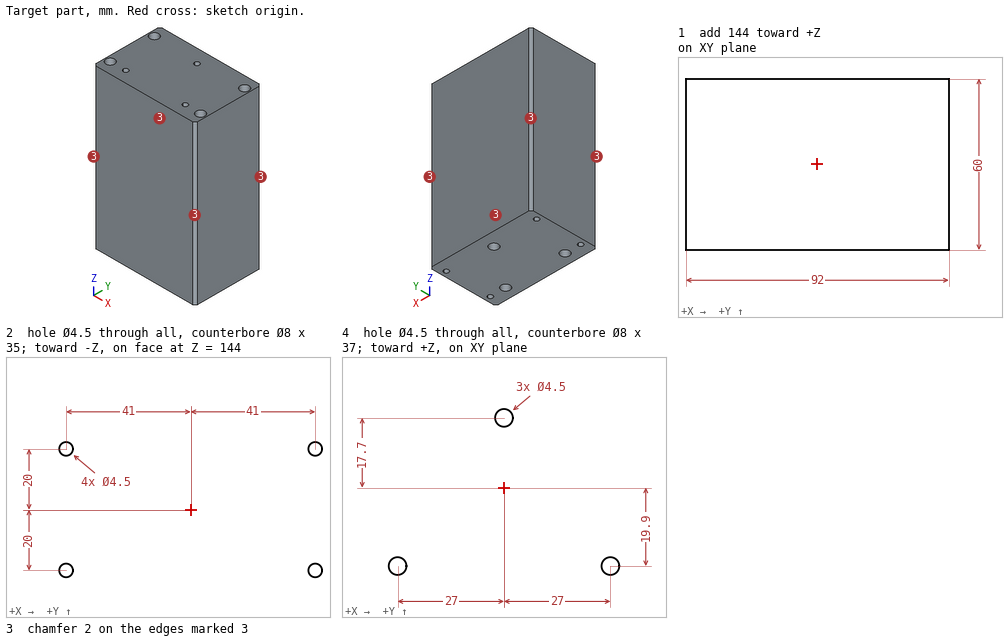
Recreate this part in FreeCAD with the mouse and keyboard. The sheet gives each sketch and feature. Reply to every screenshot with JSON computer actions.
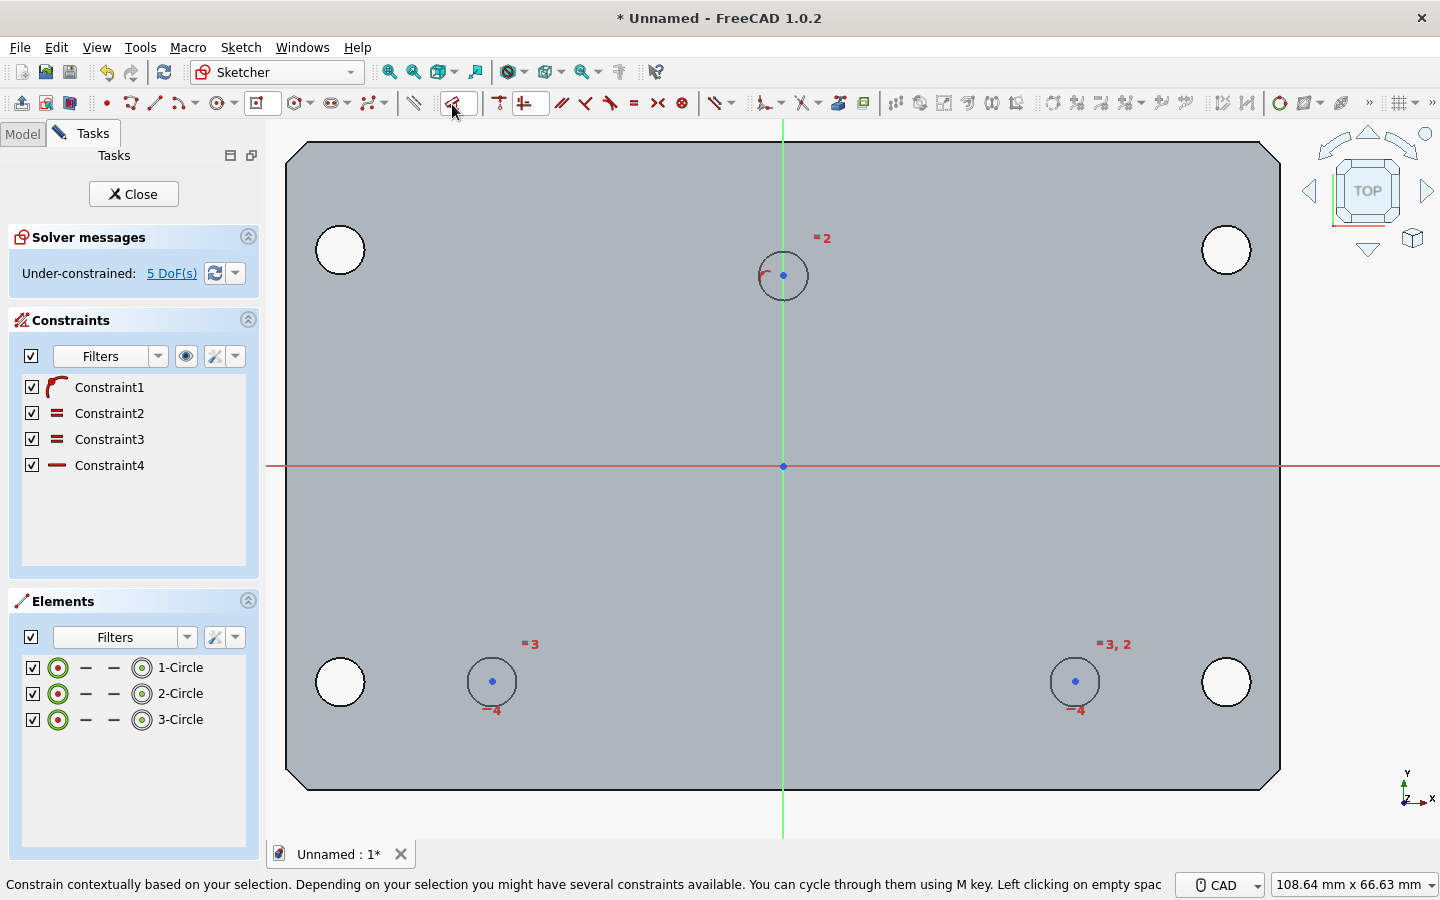
{"action": "left_click", "coordinate": [801, 259]}
{"action": "left_click", "coordinate": [824, 237]}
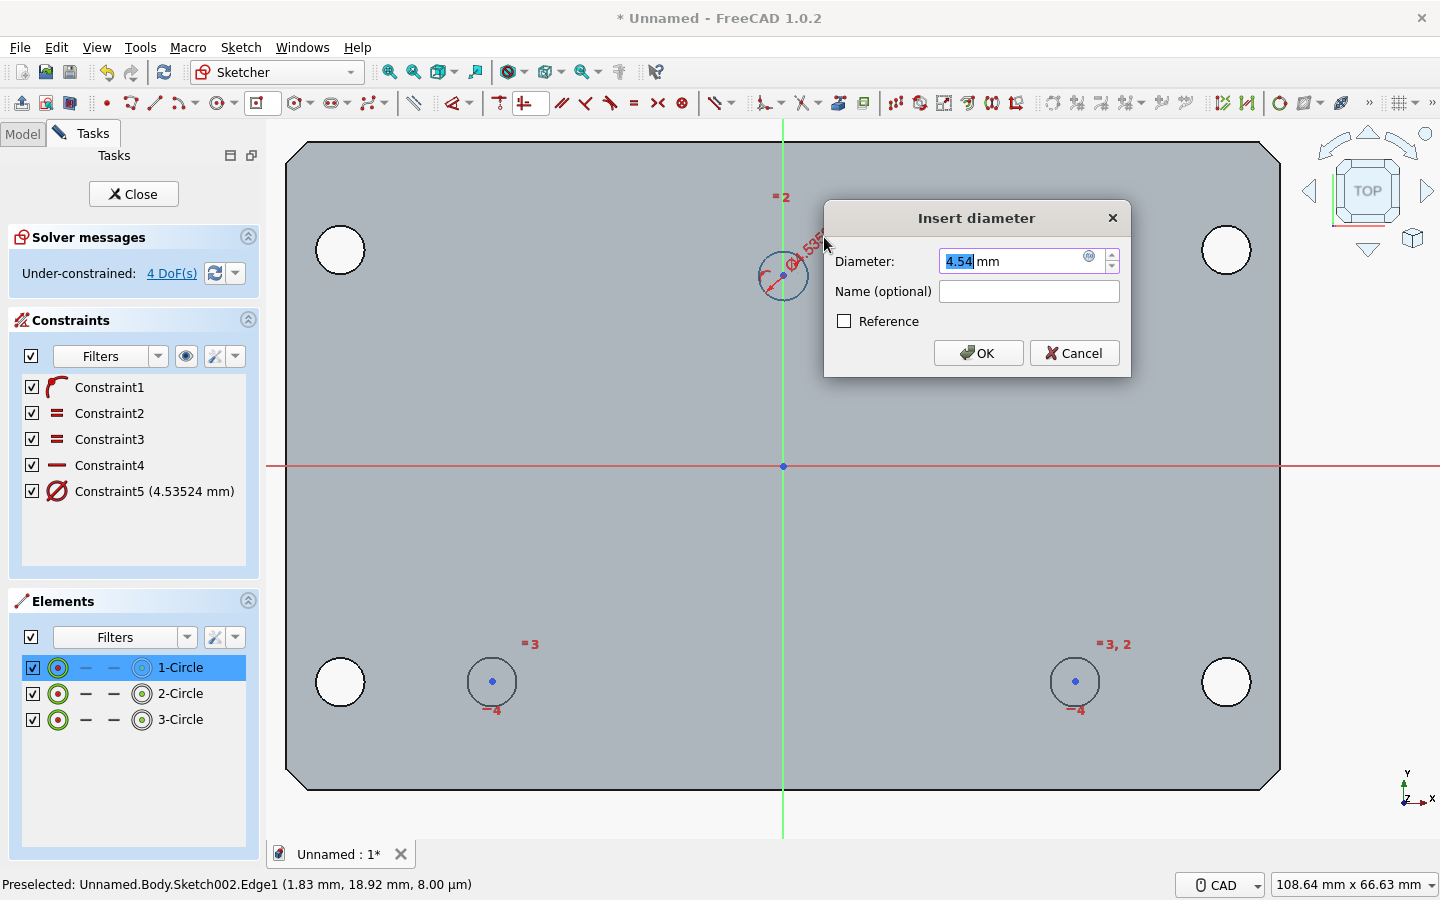
{"action": "type", "text": "4.5"}
{"action": "key", "text": "Return"}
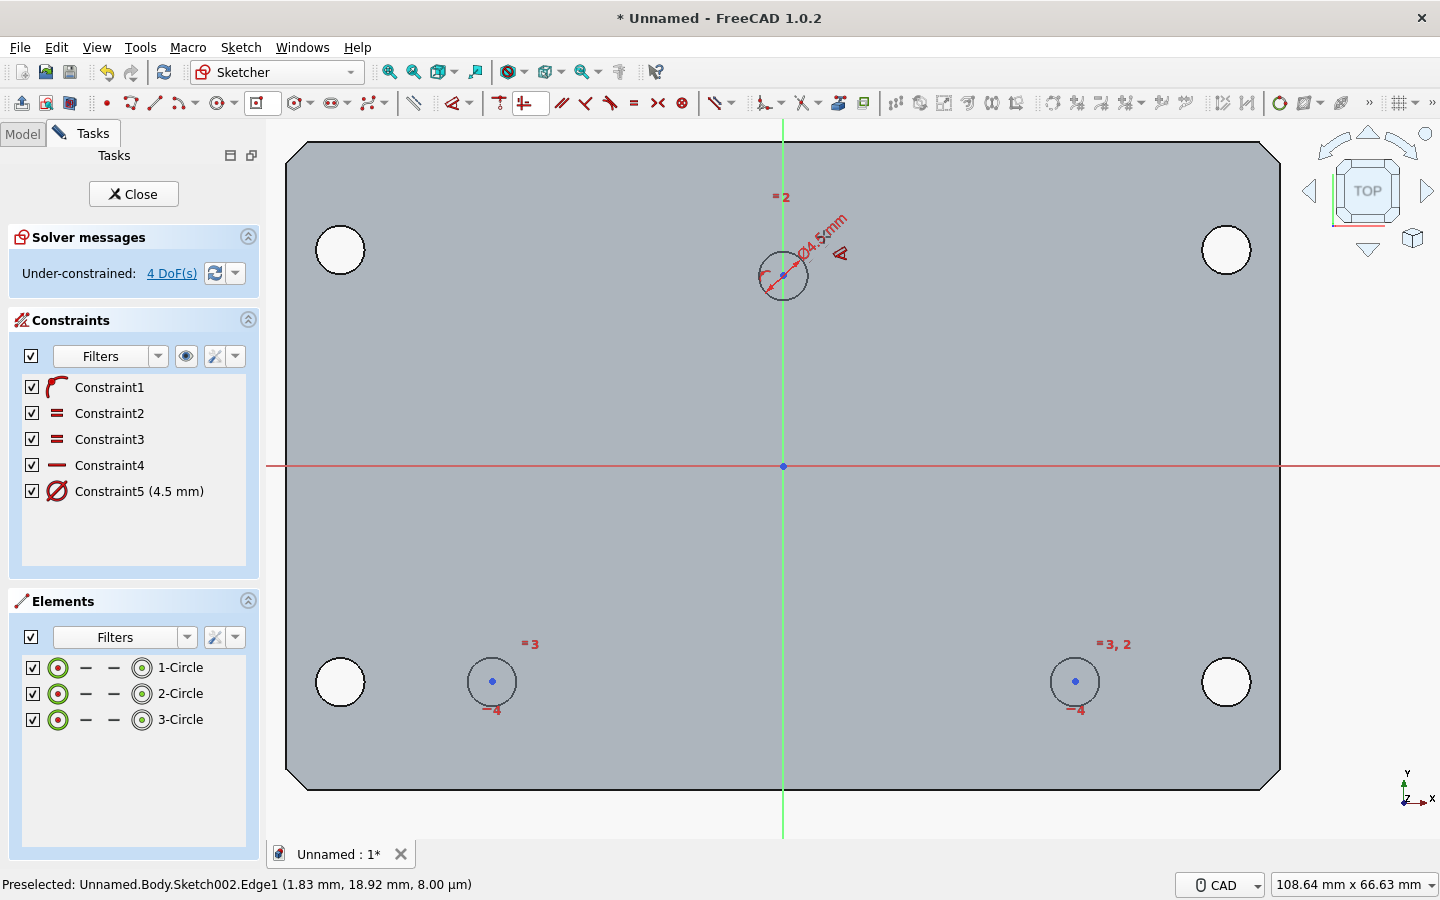
{"action": "left_click", "coordinate": [1075, 682]}
{"action": "left_click", "coordinate": [929, 716]}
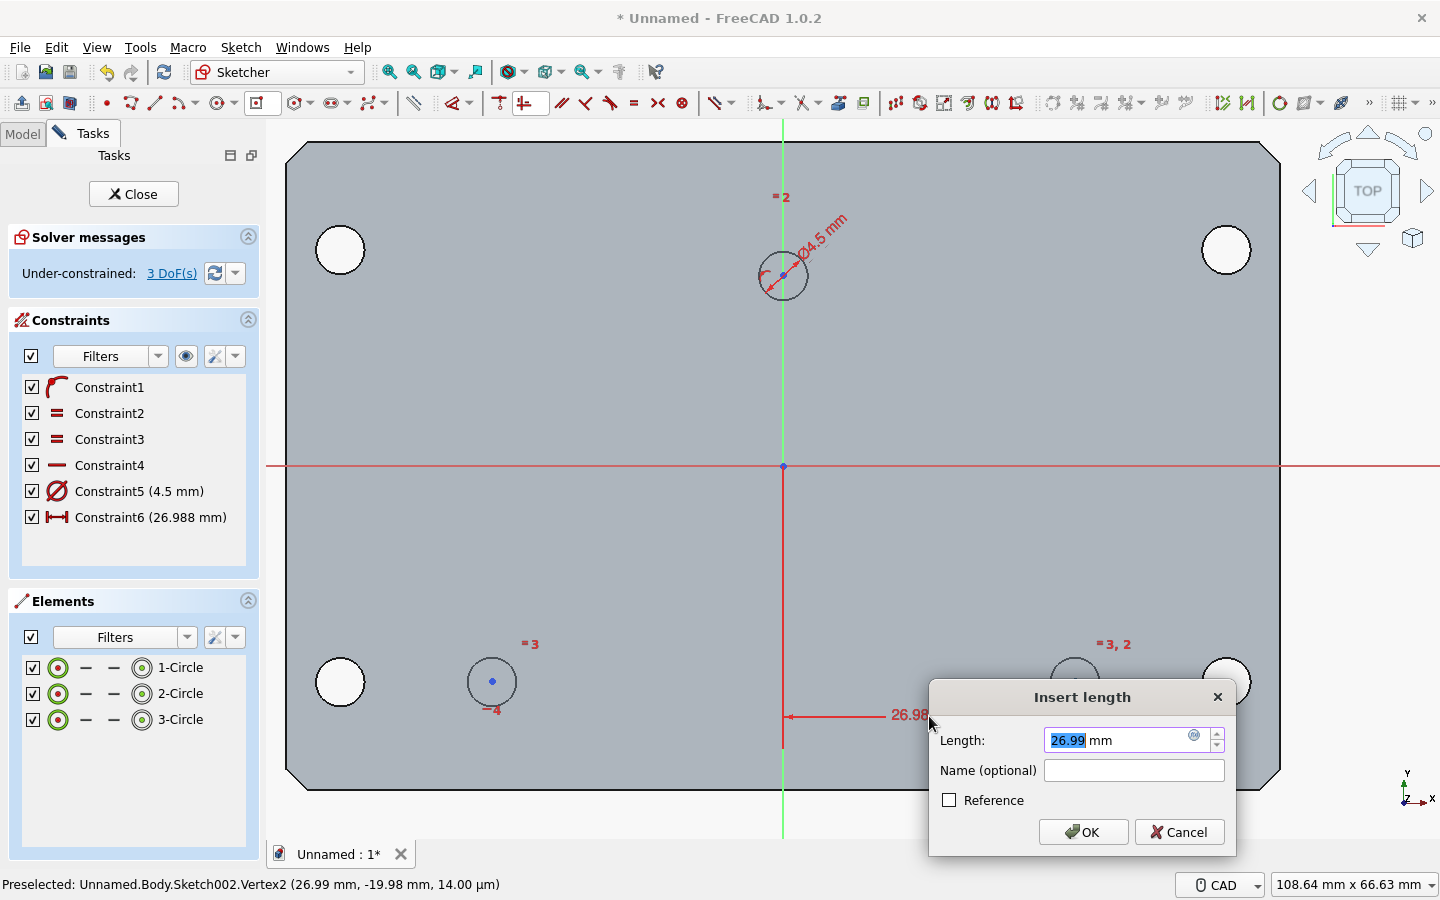
{"action": "type", "text": "27"}
{"action": "key", "text": "Return"}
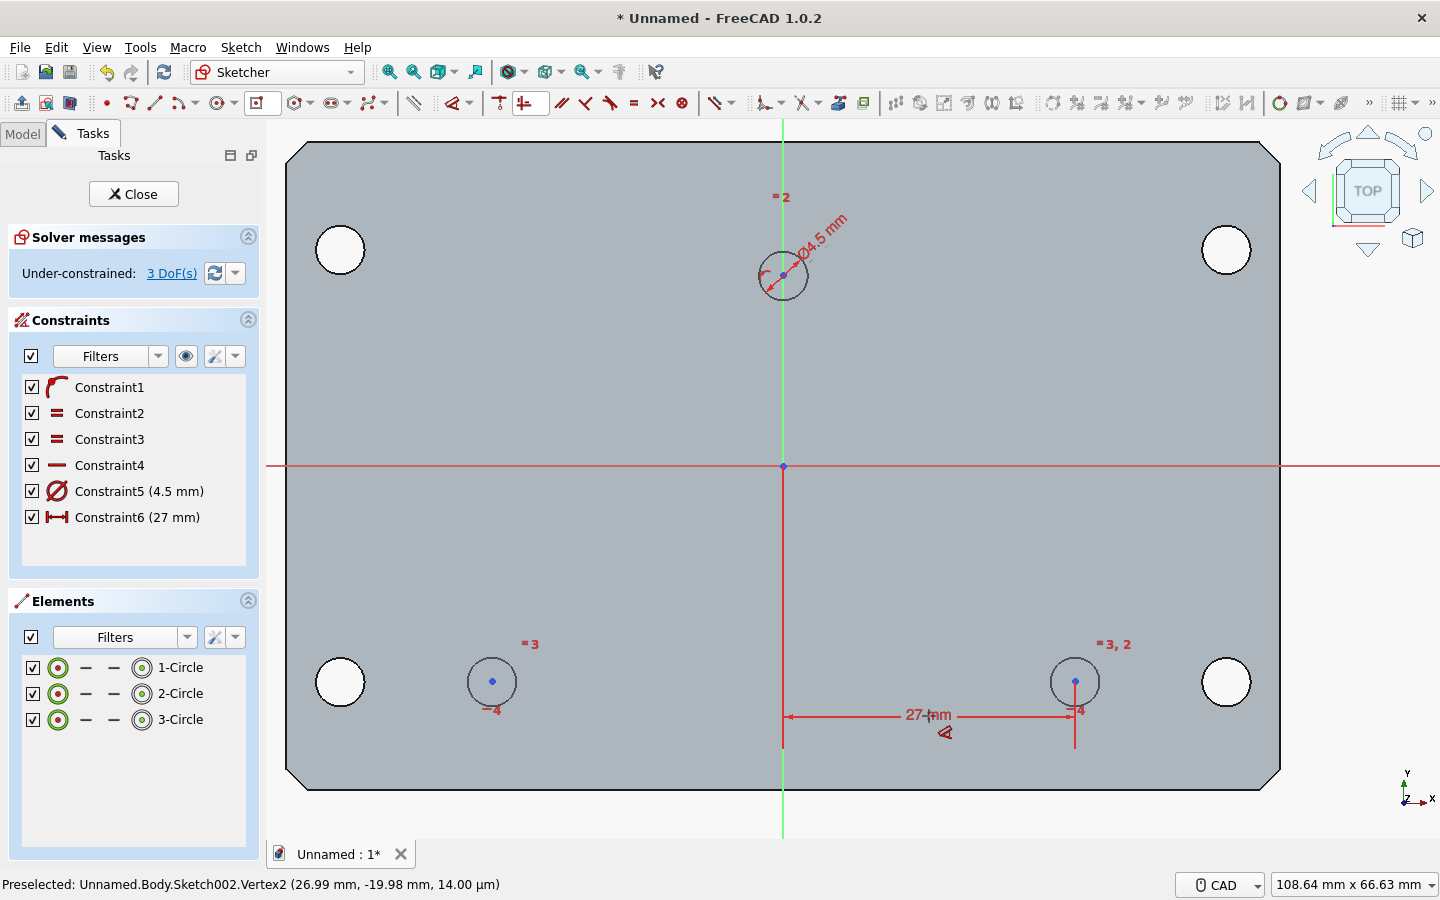
{"action": "left_click", "coordinate": [492, 682]}
{"action": "left_click", "coordinate": [638, 716]}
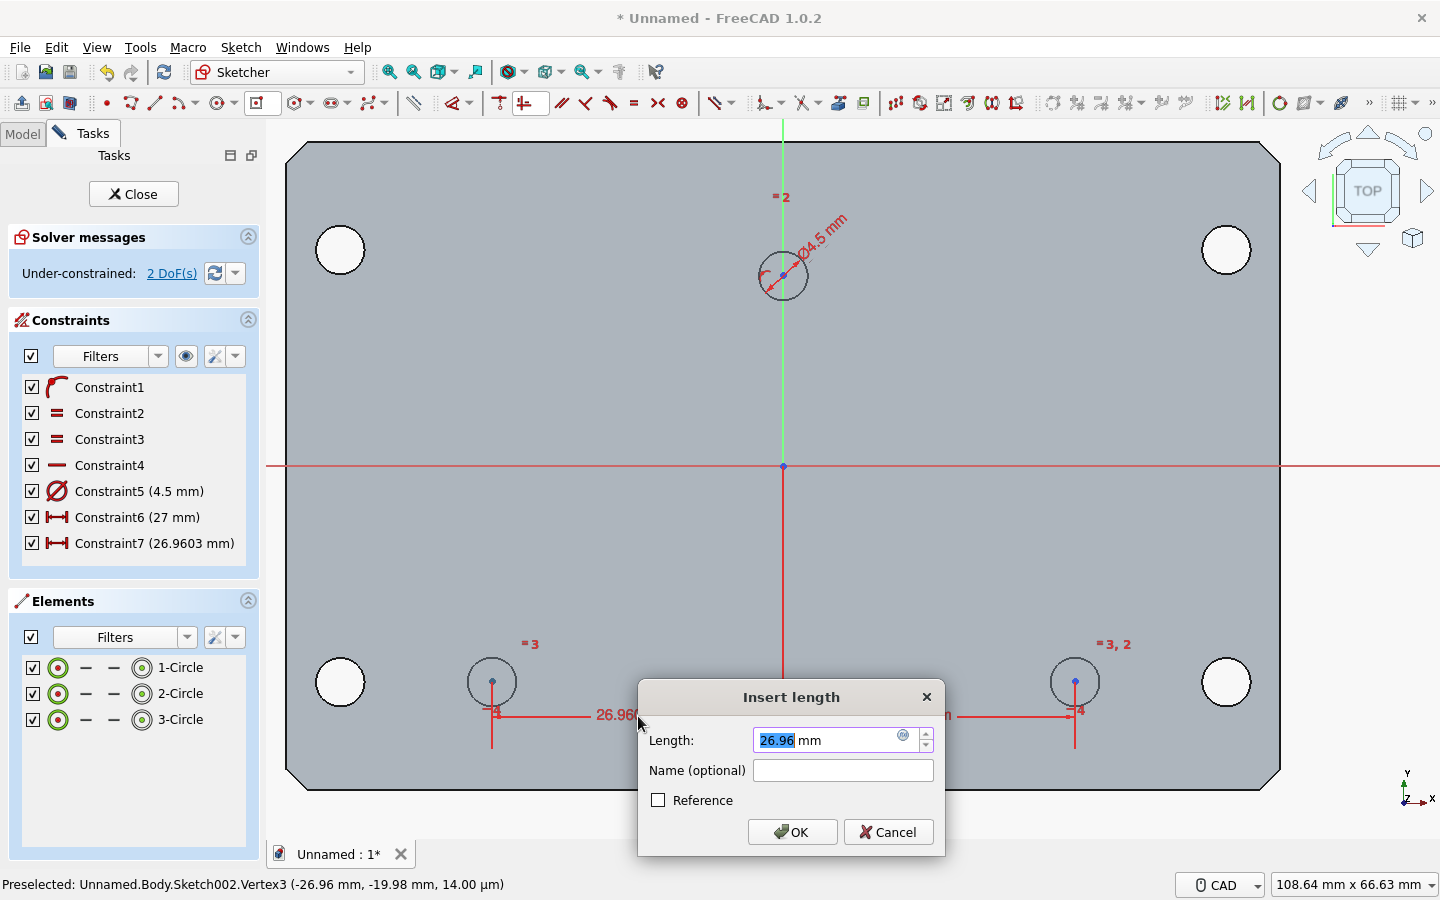
{"action": "type", "text": "27"}
{"action": "key", "text": "Return"}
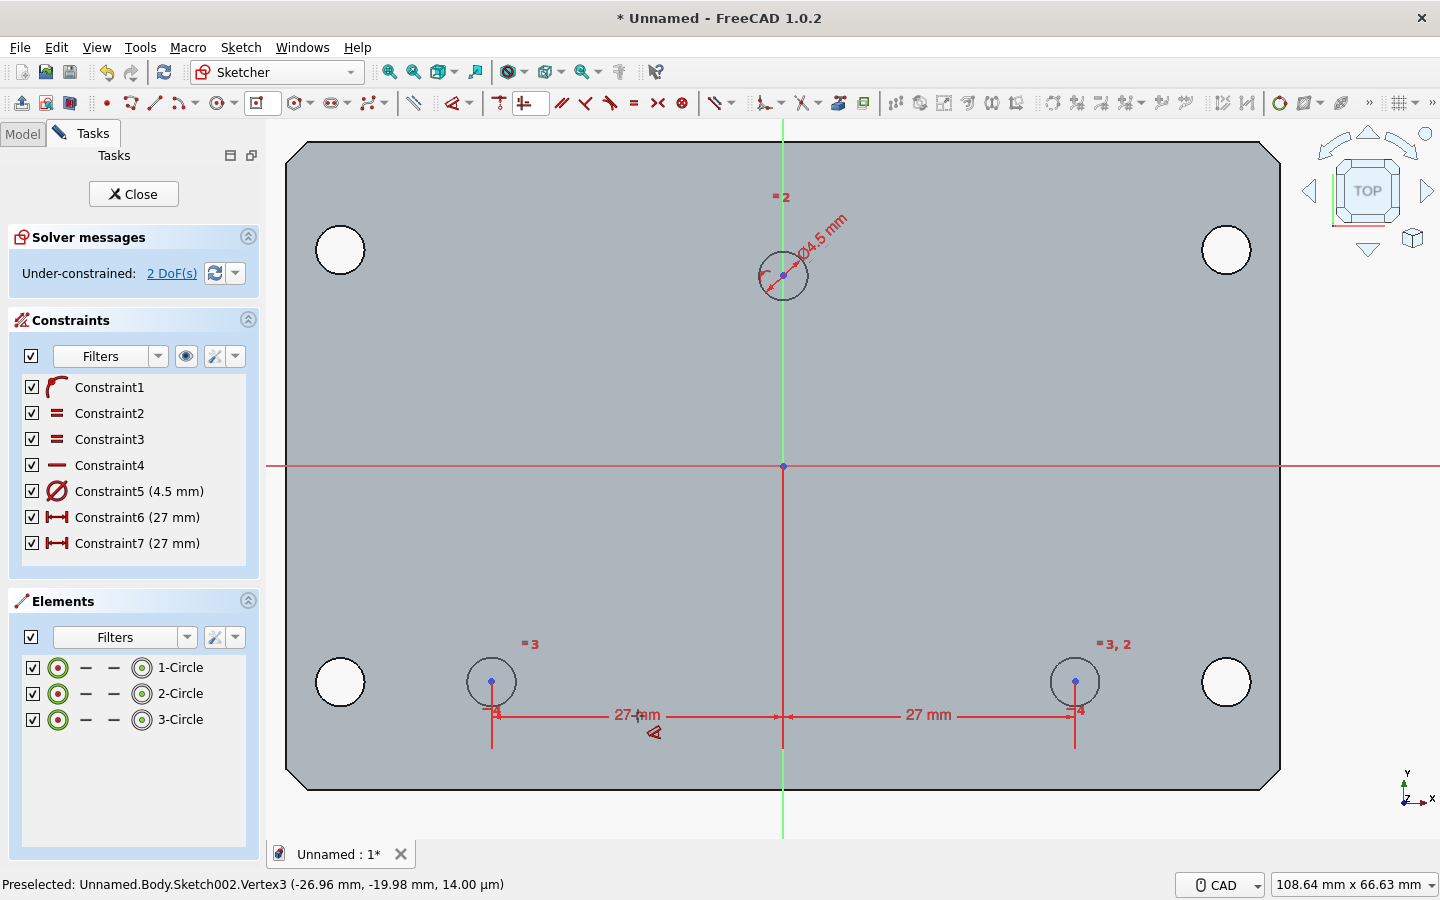
{"action": "left_click", "coordinate": [783, 276]}
{"action": "left_click", "coordinate": [817, 371]}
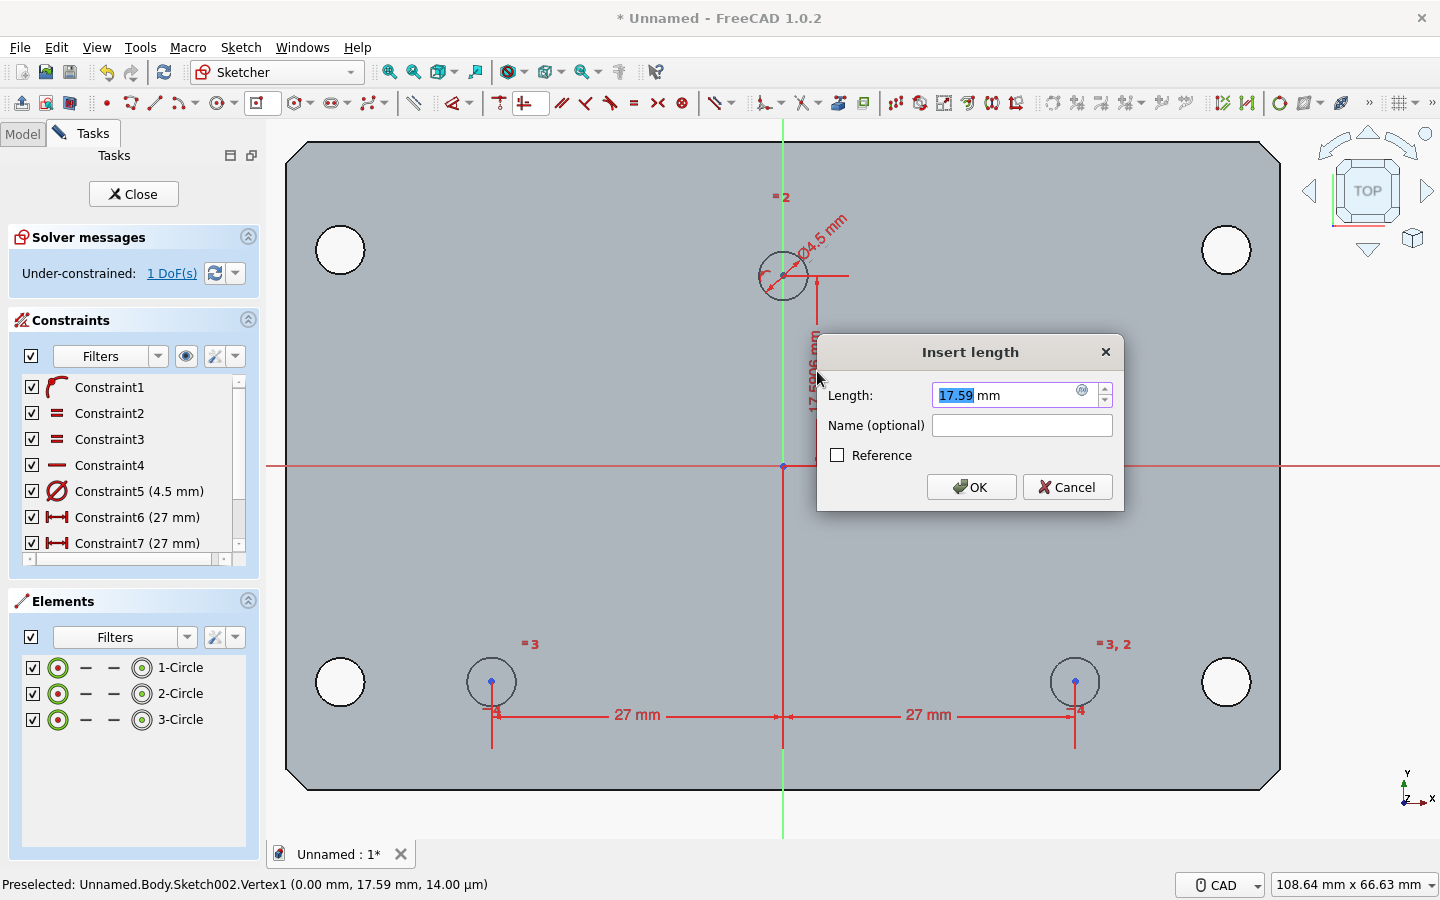
{"action": "type", "text": "17.7"}
{"action": "key", "text": "Return"}